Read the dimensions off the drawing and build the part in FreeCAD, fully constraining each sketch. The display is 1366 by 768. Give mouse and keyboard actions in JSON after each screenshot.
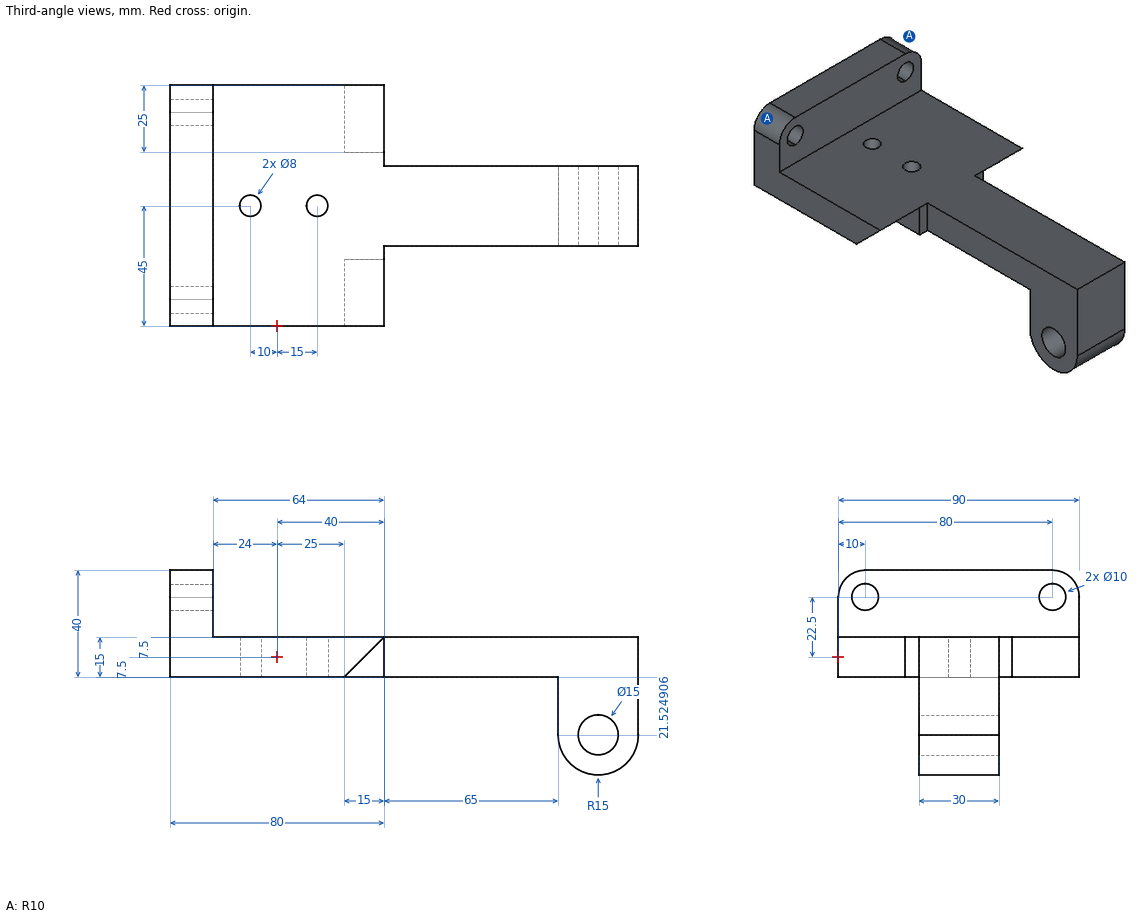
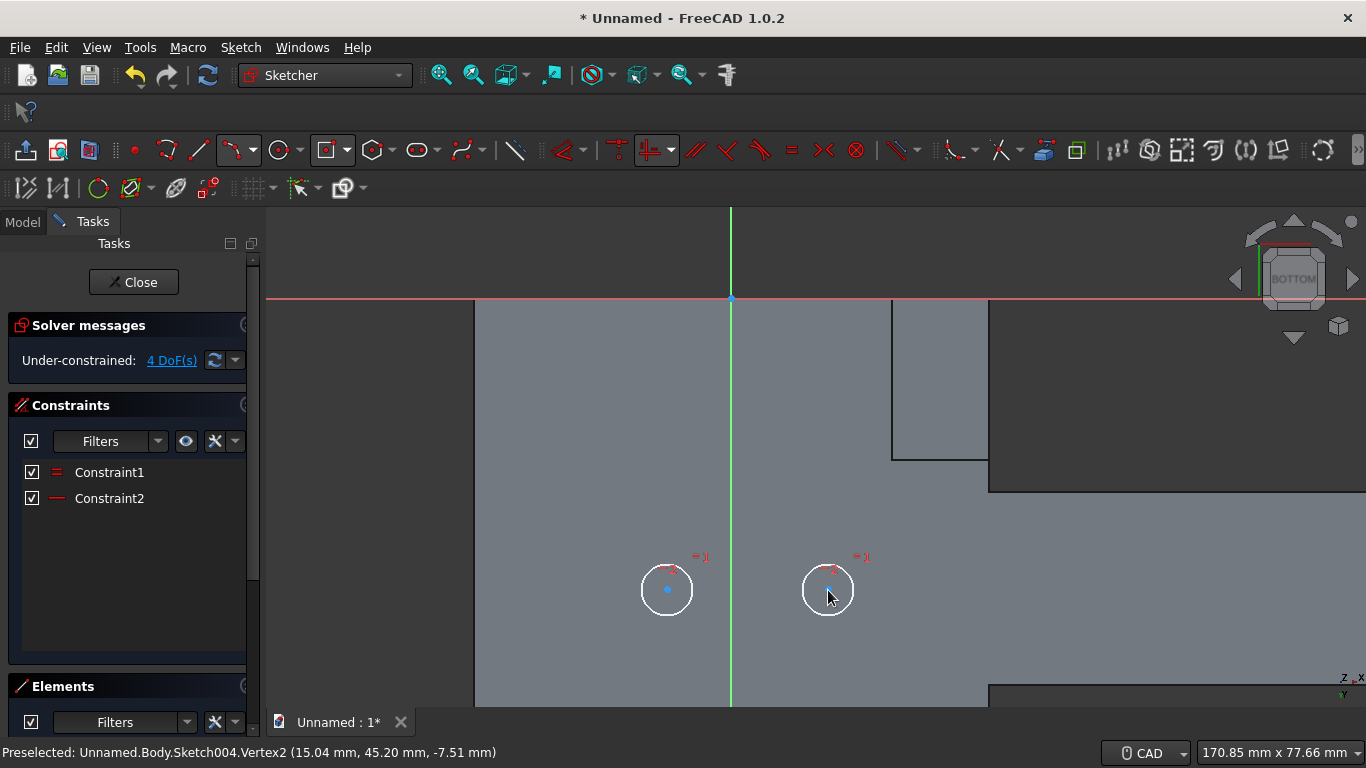
{"action": "left_click", "coordinate": [562, 150]}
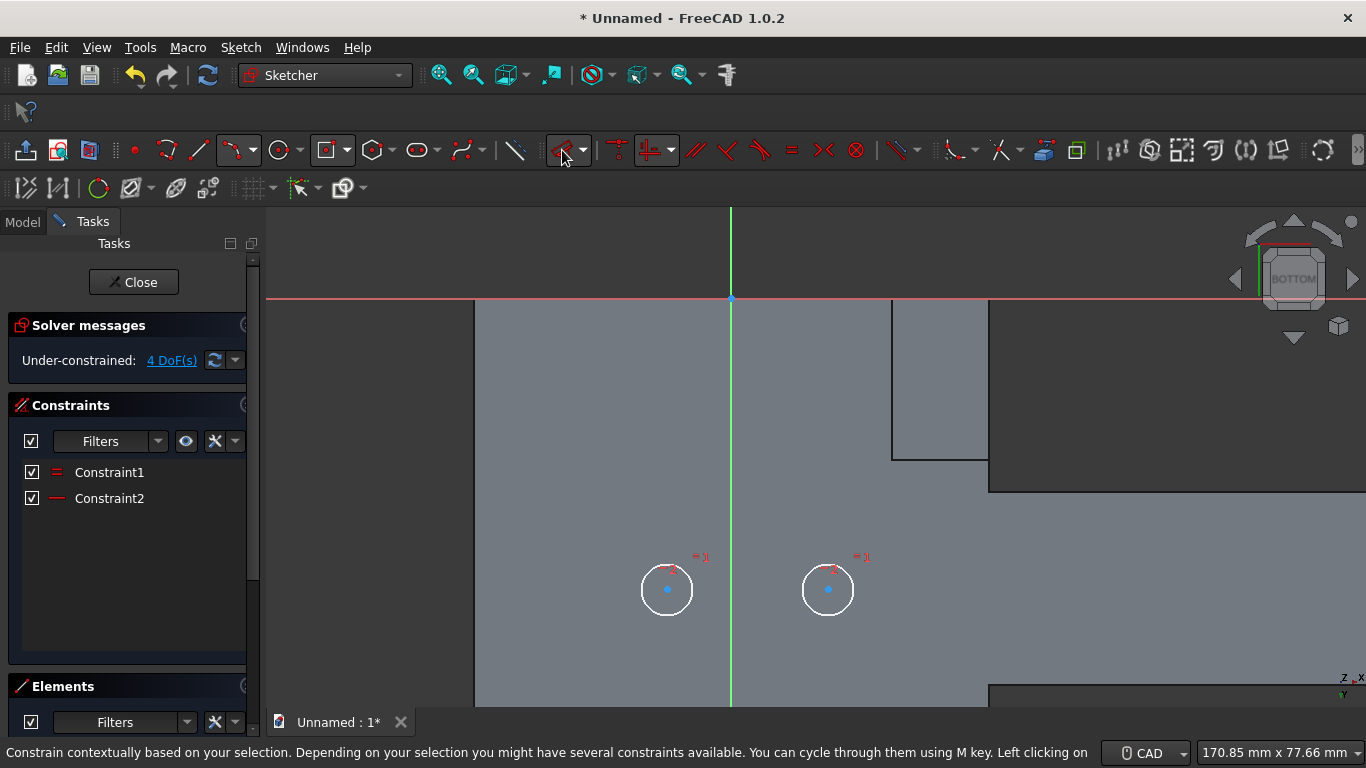
{"action": "left_click", "coordinate": [685, 572]}
{"action": "left_click", "coordinate": [708, 549]}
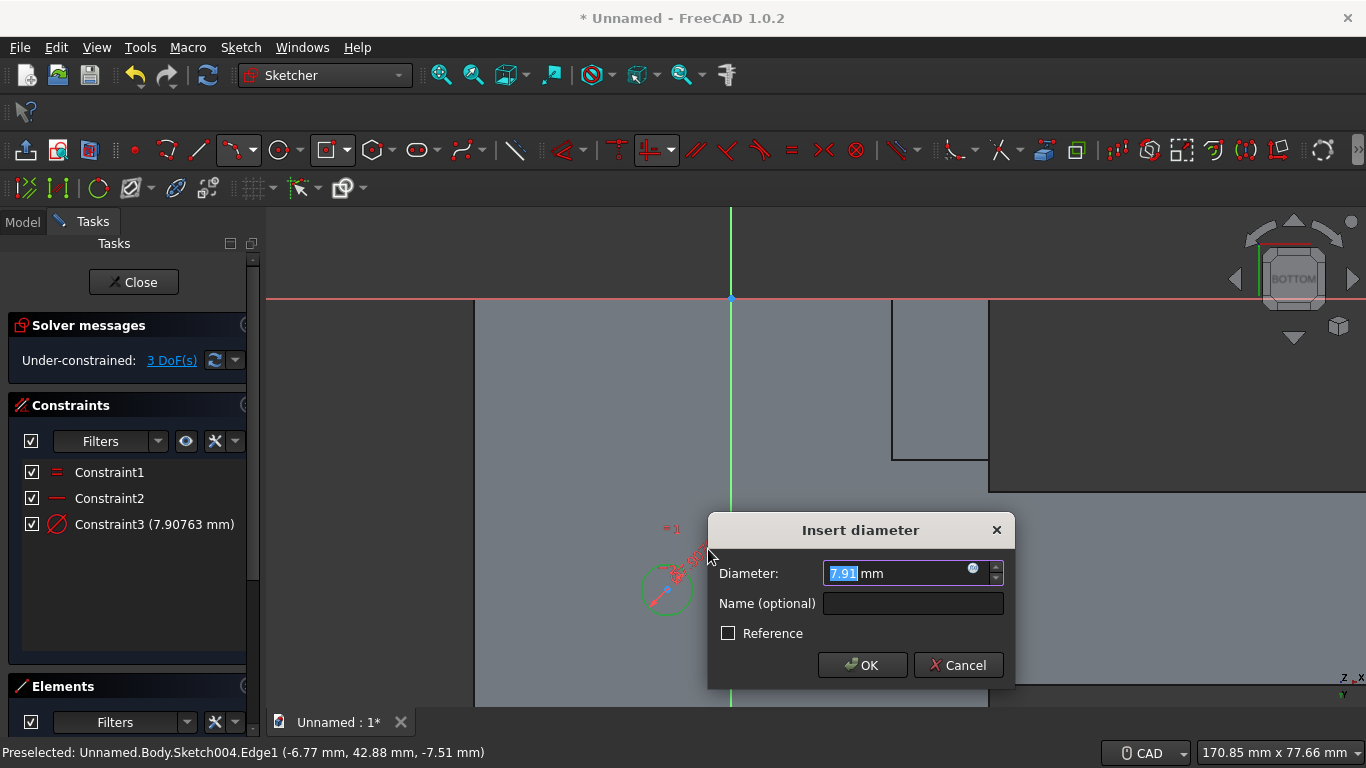
{"action": "type", "text": "8"}
{"action": "key", "text": "Return"}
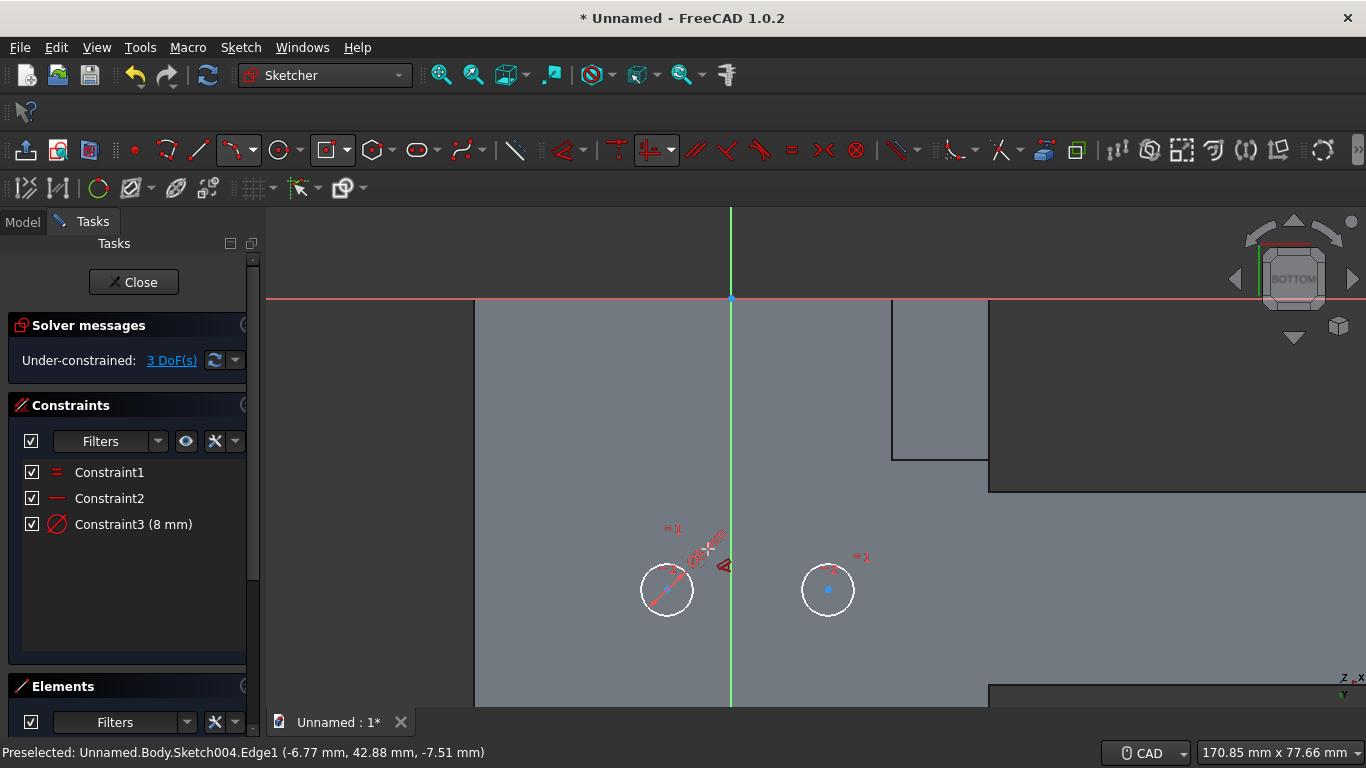
{"action": "left_click", "coordinate": [667, 590]}
{"action": "left_click", "coordinate": [699, 265]}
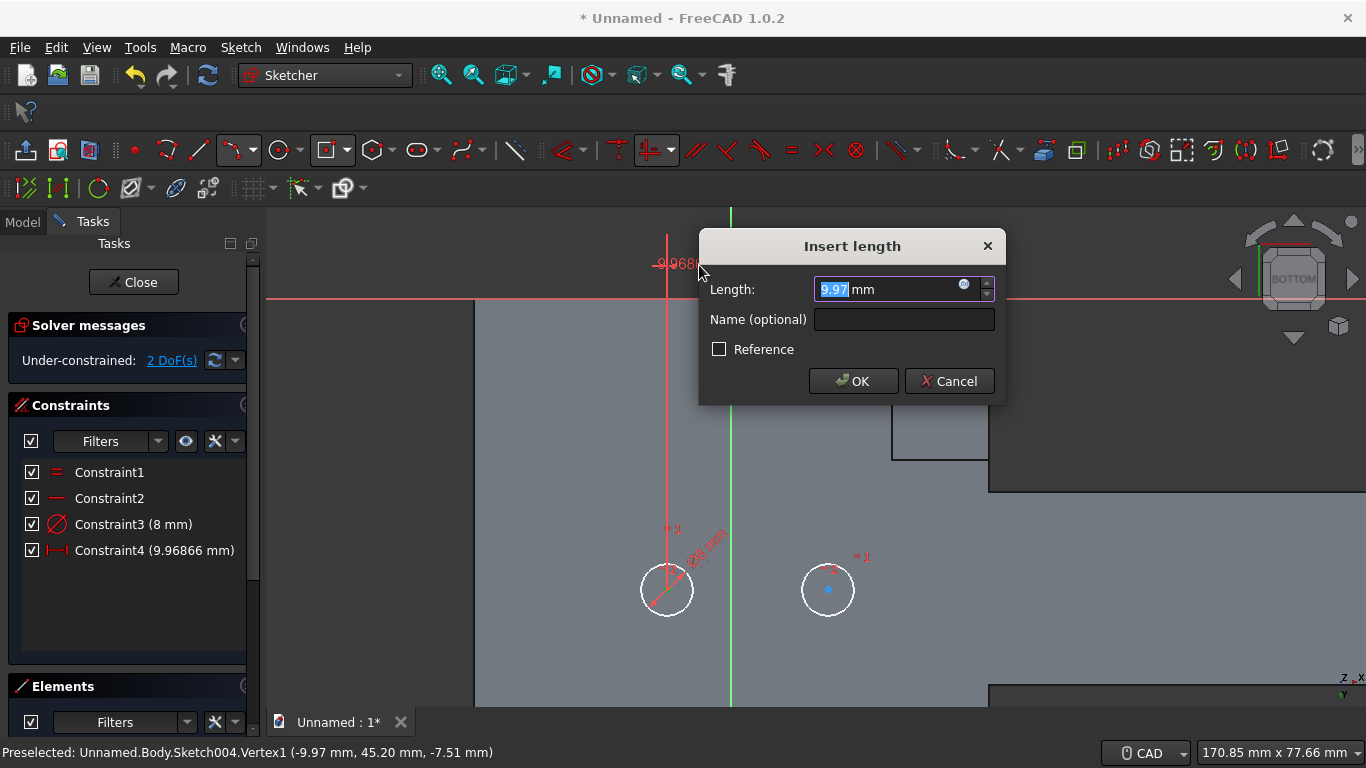
{"action": "type", "text": "10"}
{"action": "key", "text": "Return"}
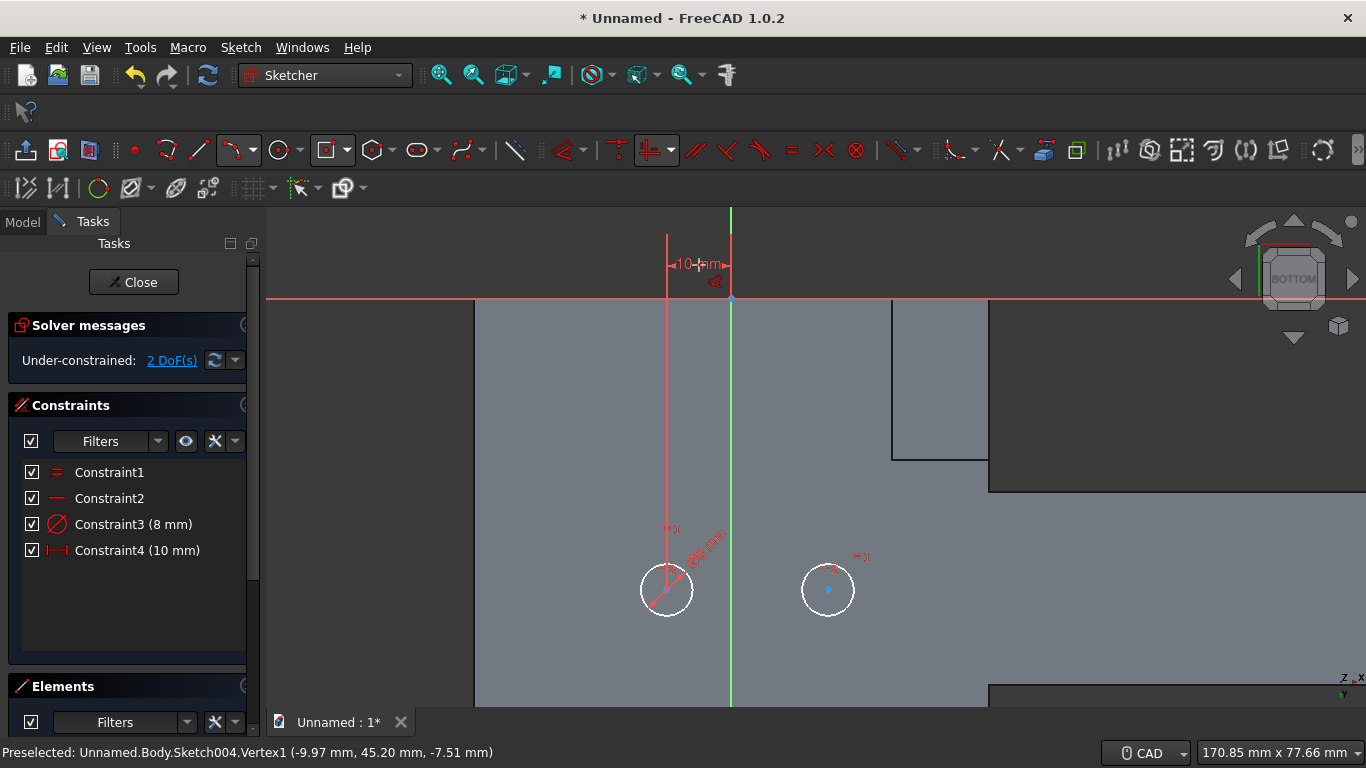
{"action": "left_click", "coordinate": [667, 590]}
{"action": "left_click", "coordinate": [633, 444]}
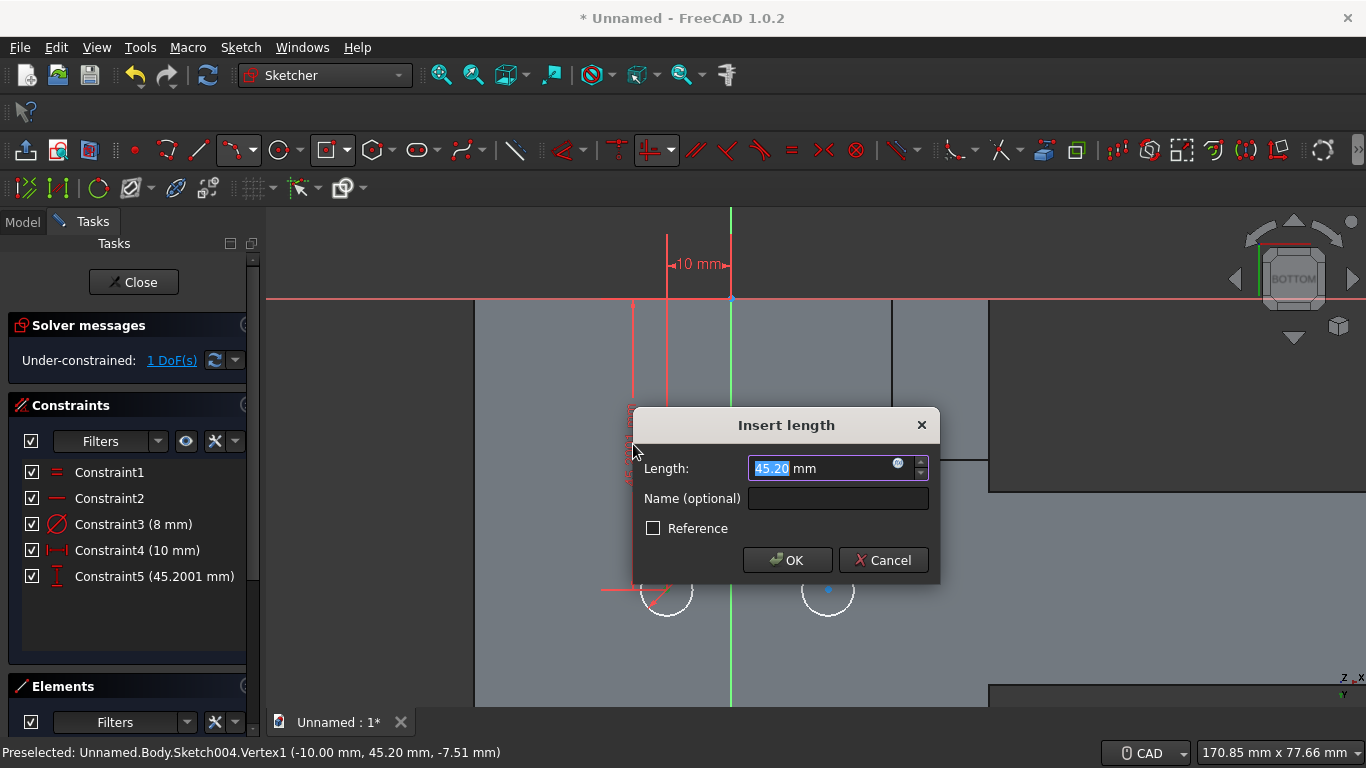
{"action": "type", "text": "45"}
{"action": "key", "text": "Return"}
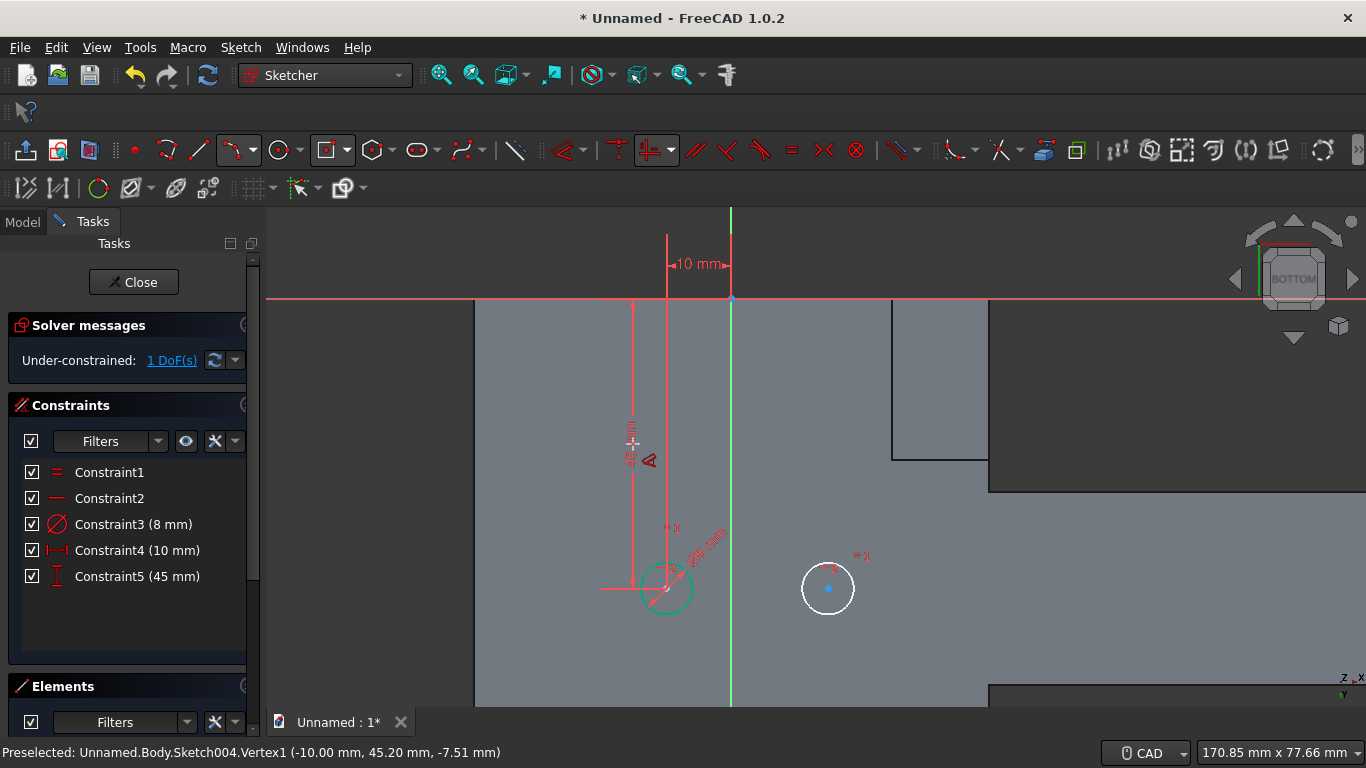
{"action": "left_click", "coordinate": [828, 589]}
{"action": "left_click", "coordinate": [780, 265]}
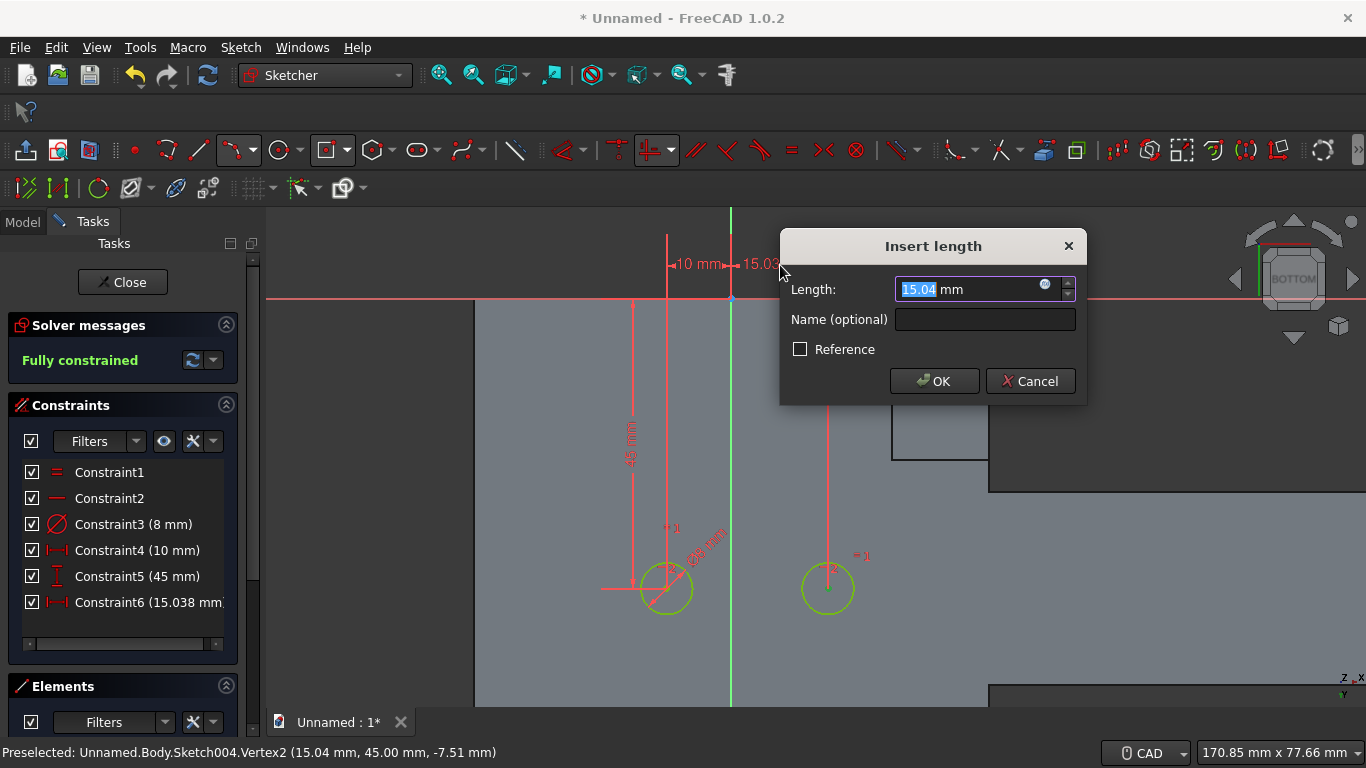
{"action": "type", "text": "15"}
{"action": "key", "text": "Return"}
{"action": "key", "text": "Escape"}